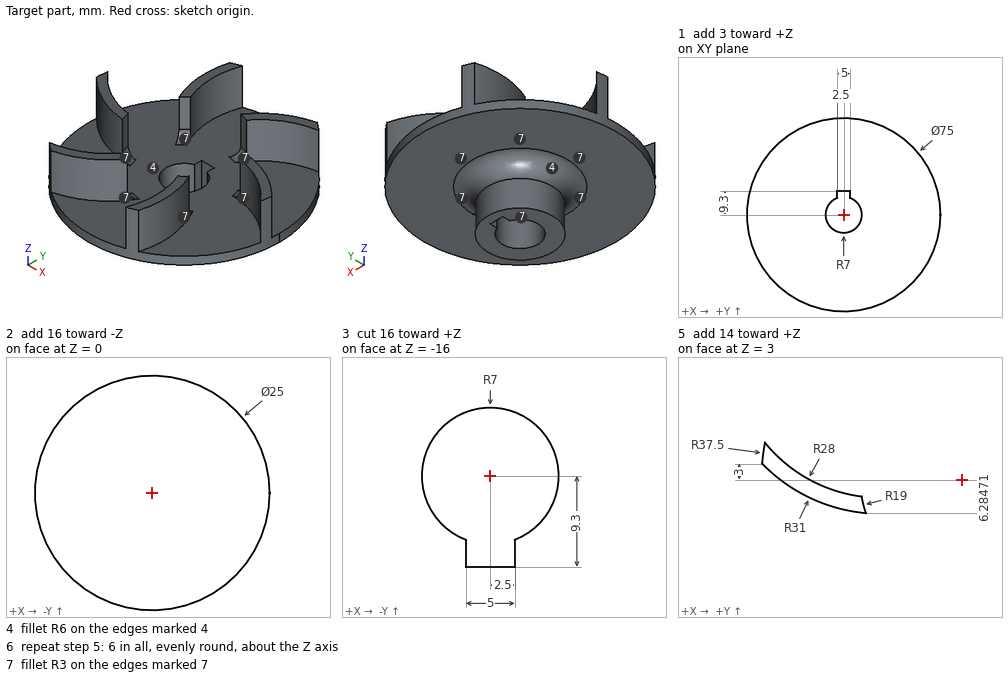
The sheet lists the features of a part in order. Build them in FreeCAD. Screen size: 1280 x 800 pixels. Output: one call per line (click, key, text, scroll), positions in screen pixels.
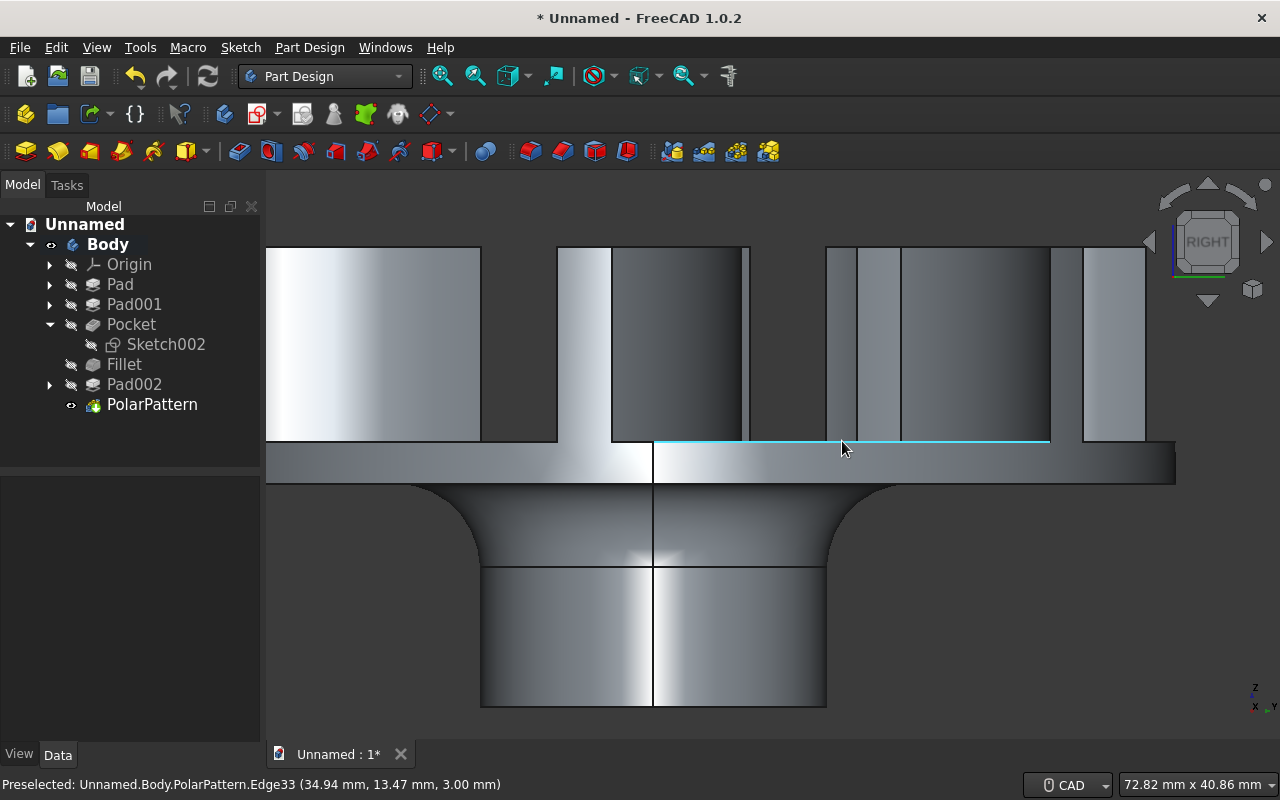
key(v)
key(f)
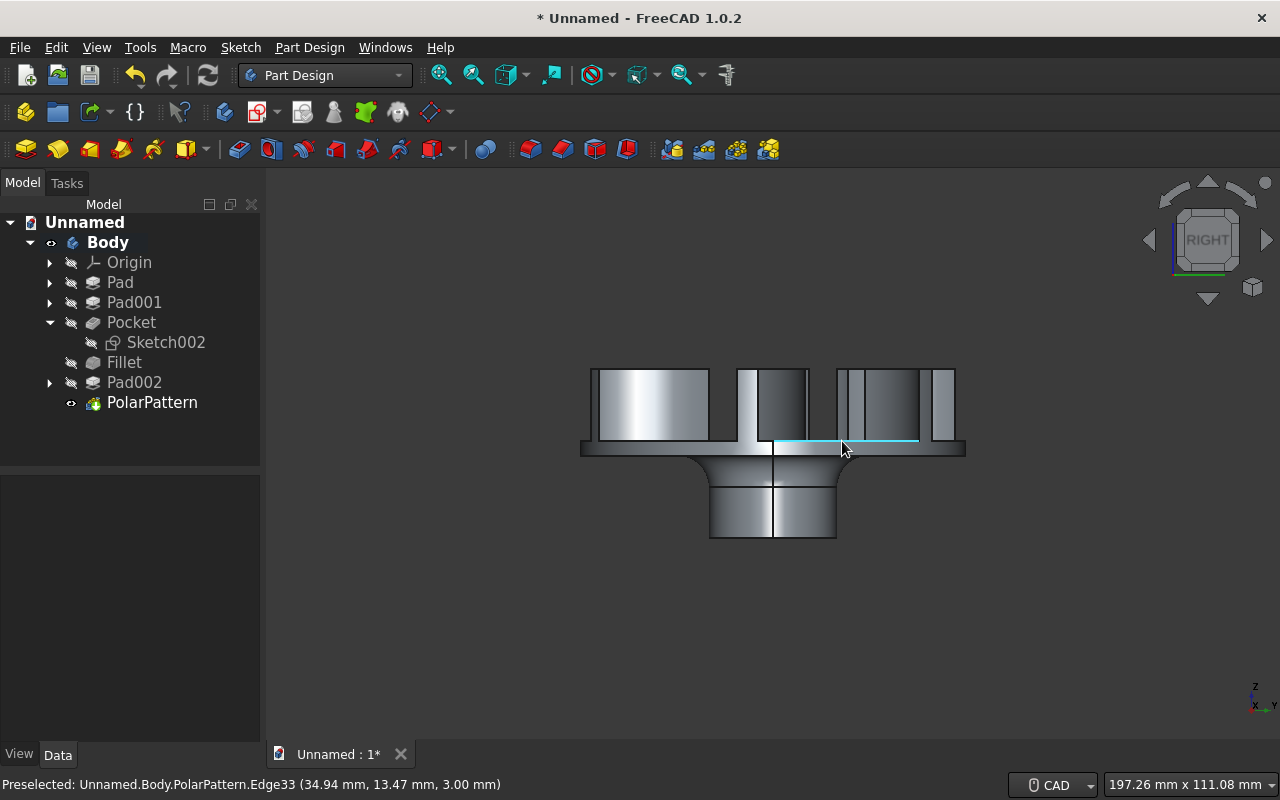
key(5)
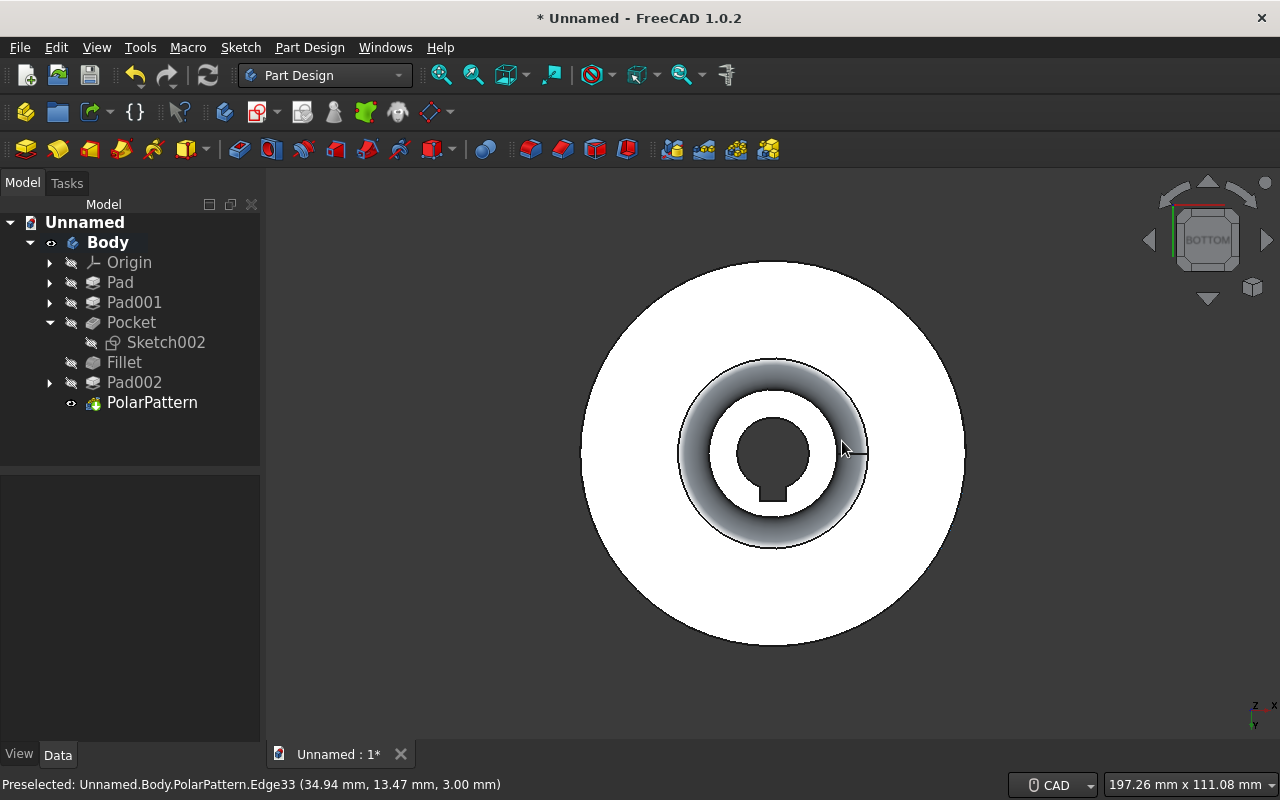
scroll(705, 522, up, 5)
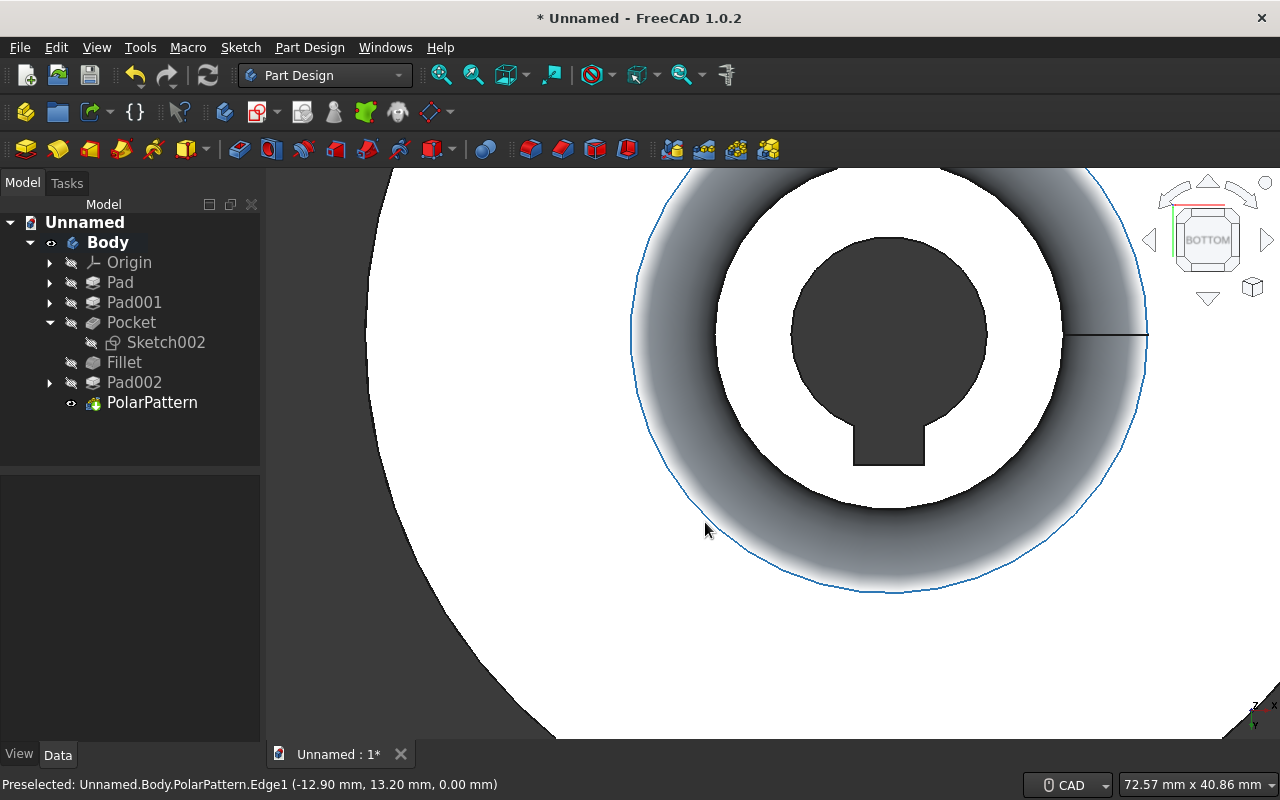
key(v)
key(f)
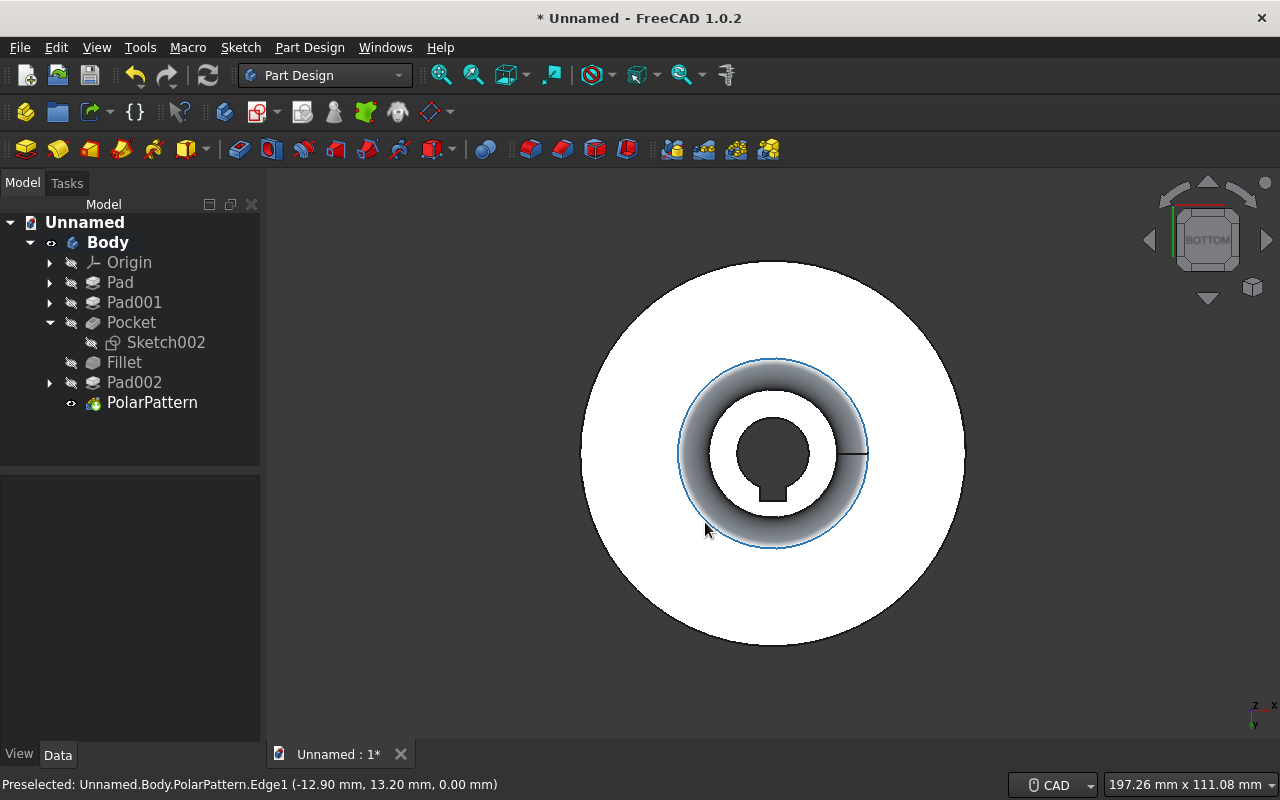
key(4)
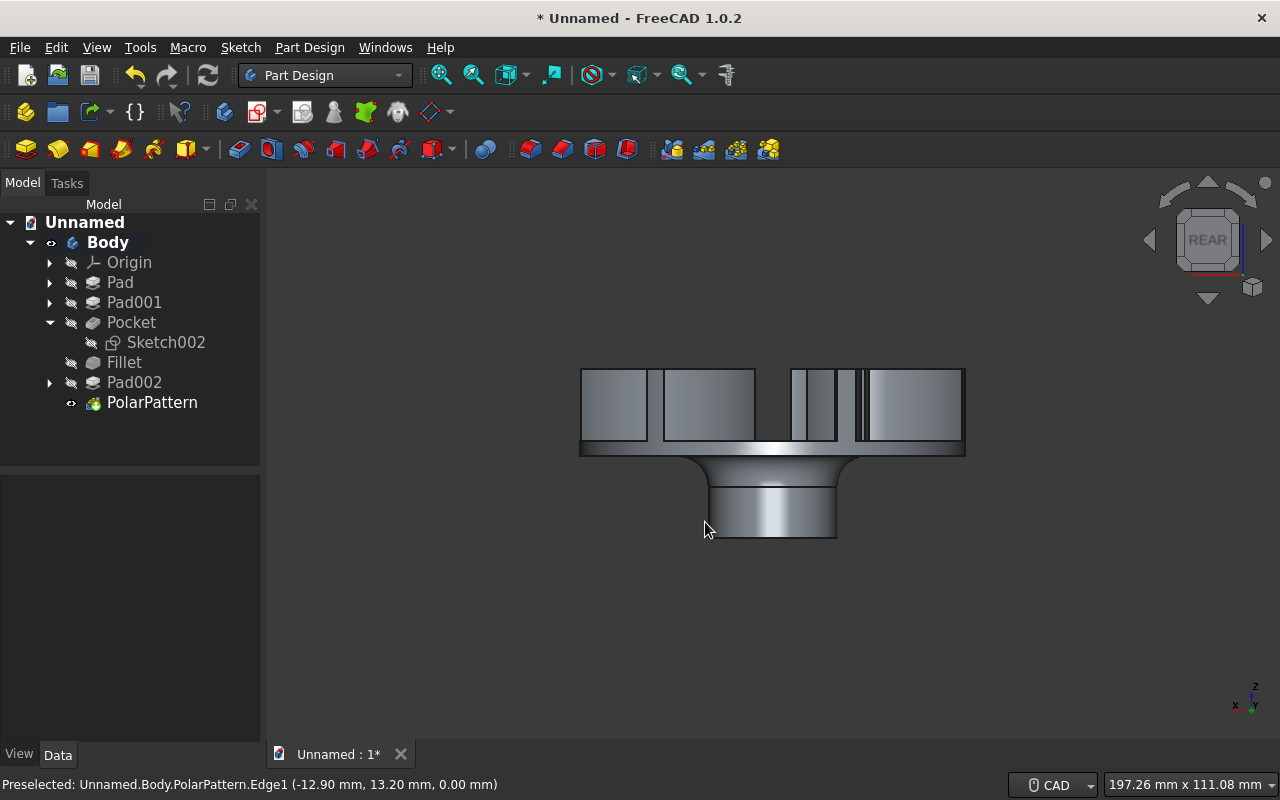
key(v)
key(f)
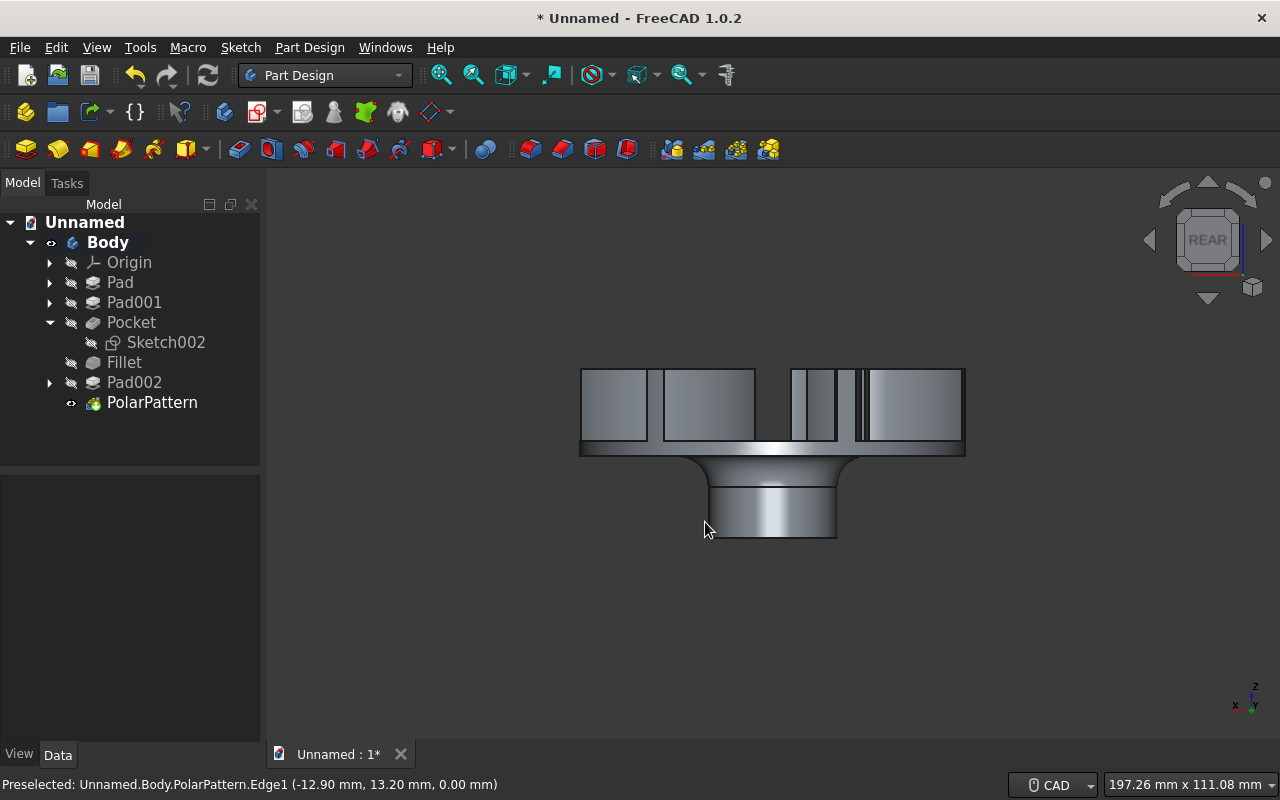
scroll(841, 440, up, 5)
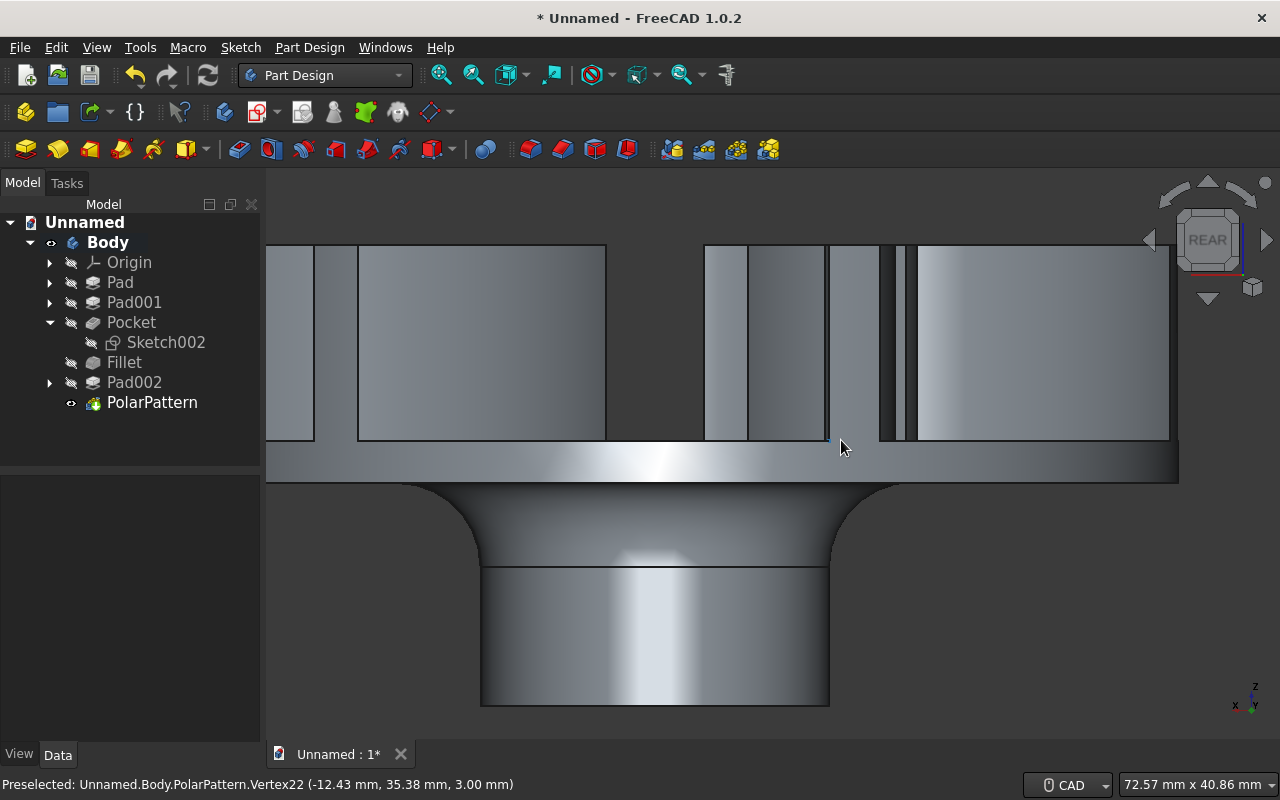
click(442, 76)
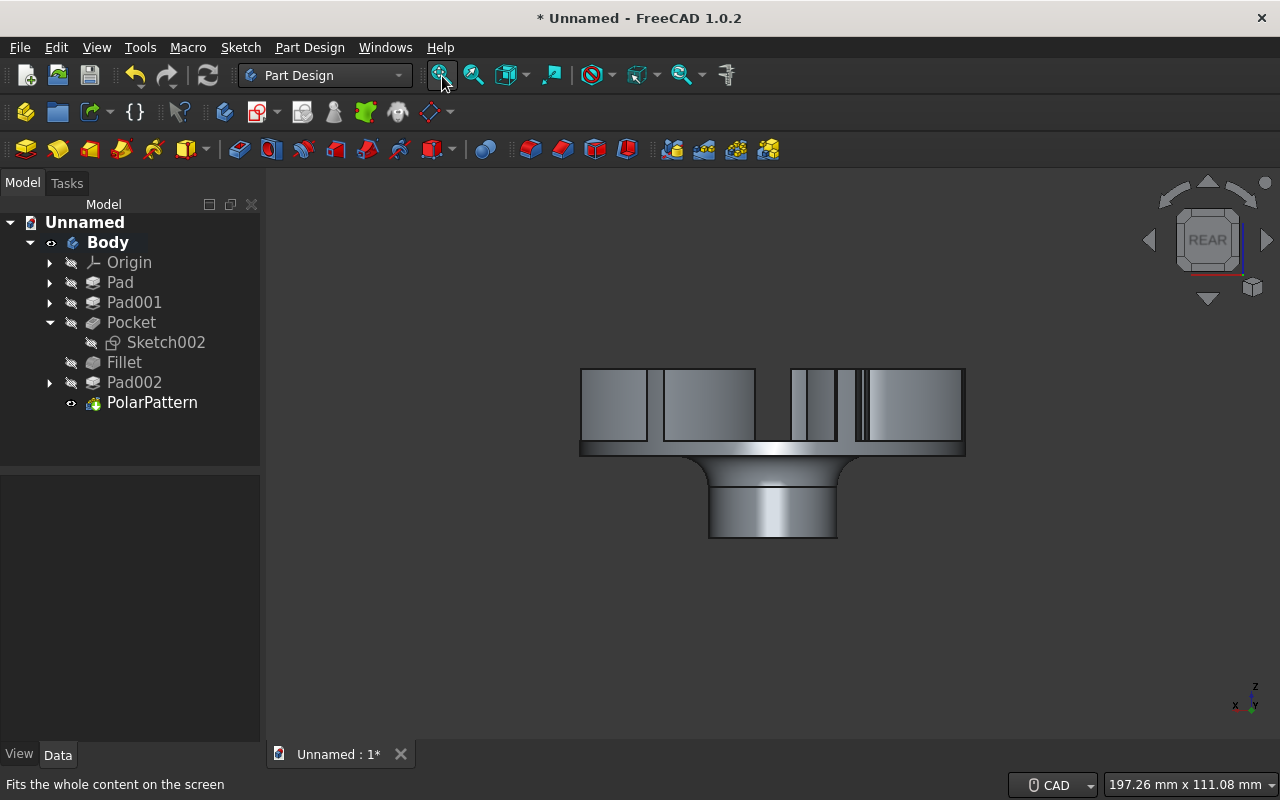
key(6)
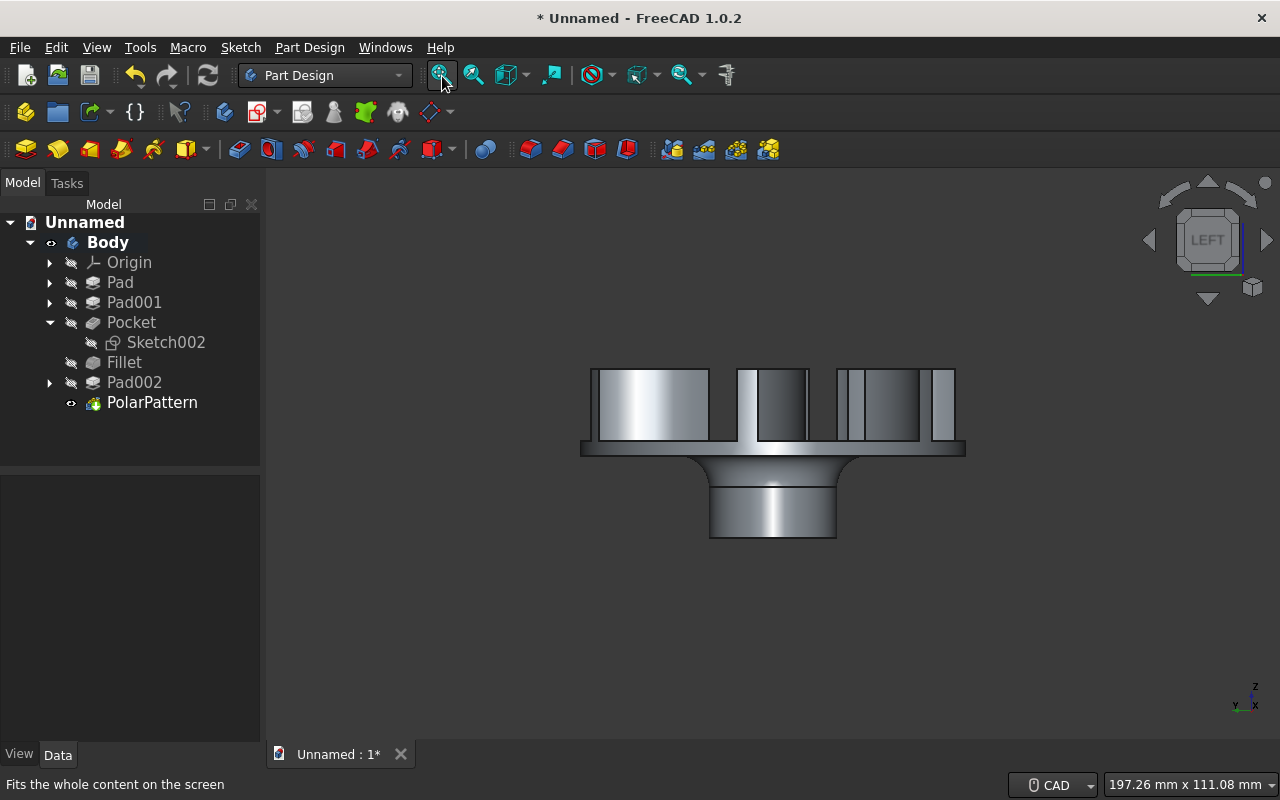
key(v)
key(f)